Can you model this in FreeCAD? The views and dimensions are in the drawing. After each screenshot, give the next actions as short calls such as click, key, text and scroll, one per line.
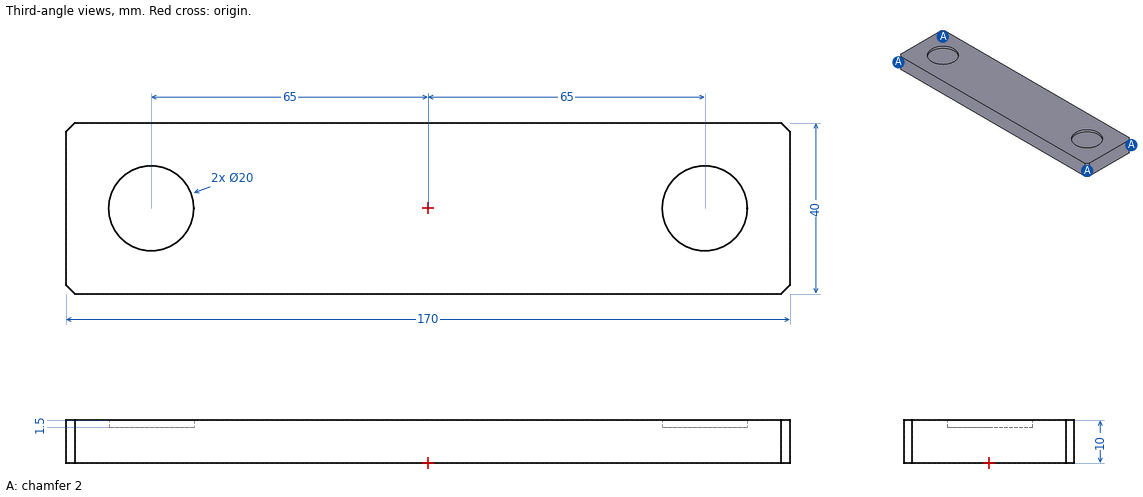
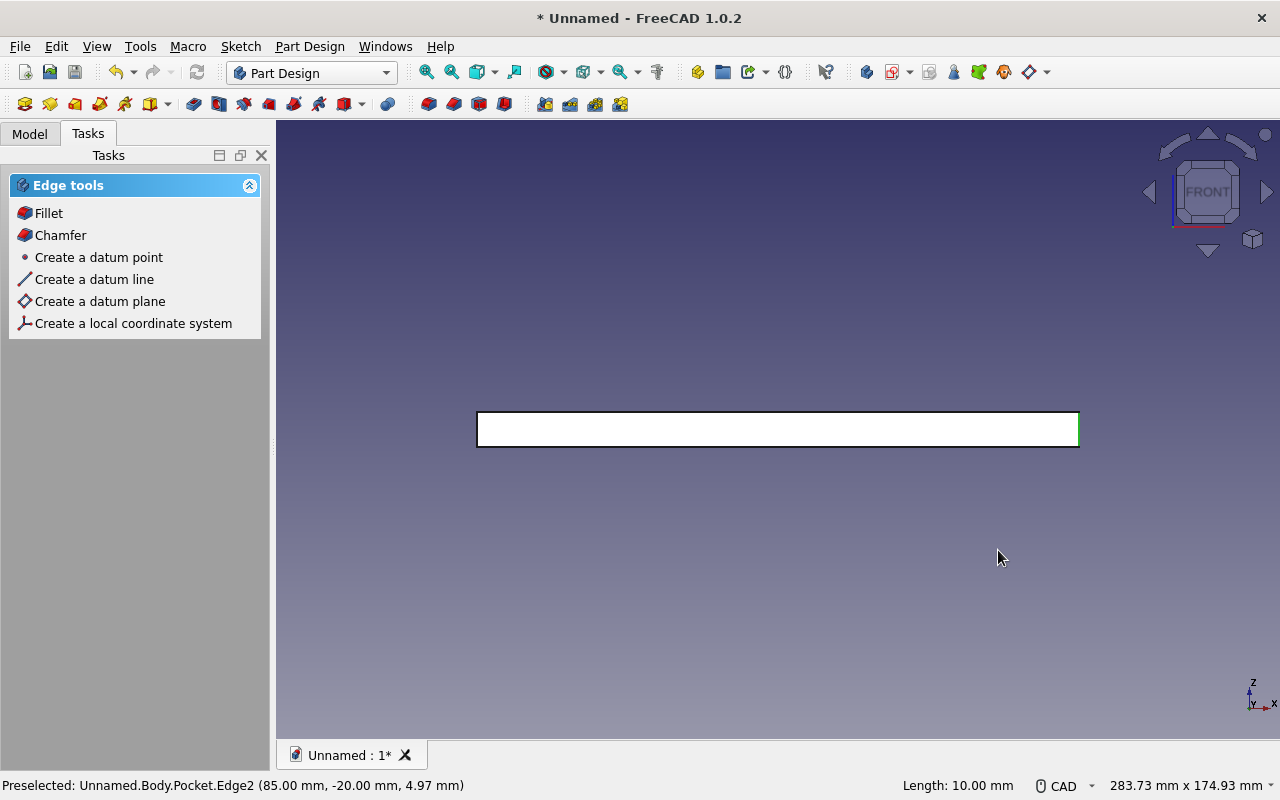
click(477, 428, ctrl)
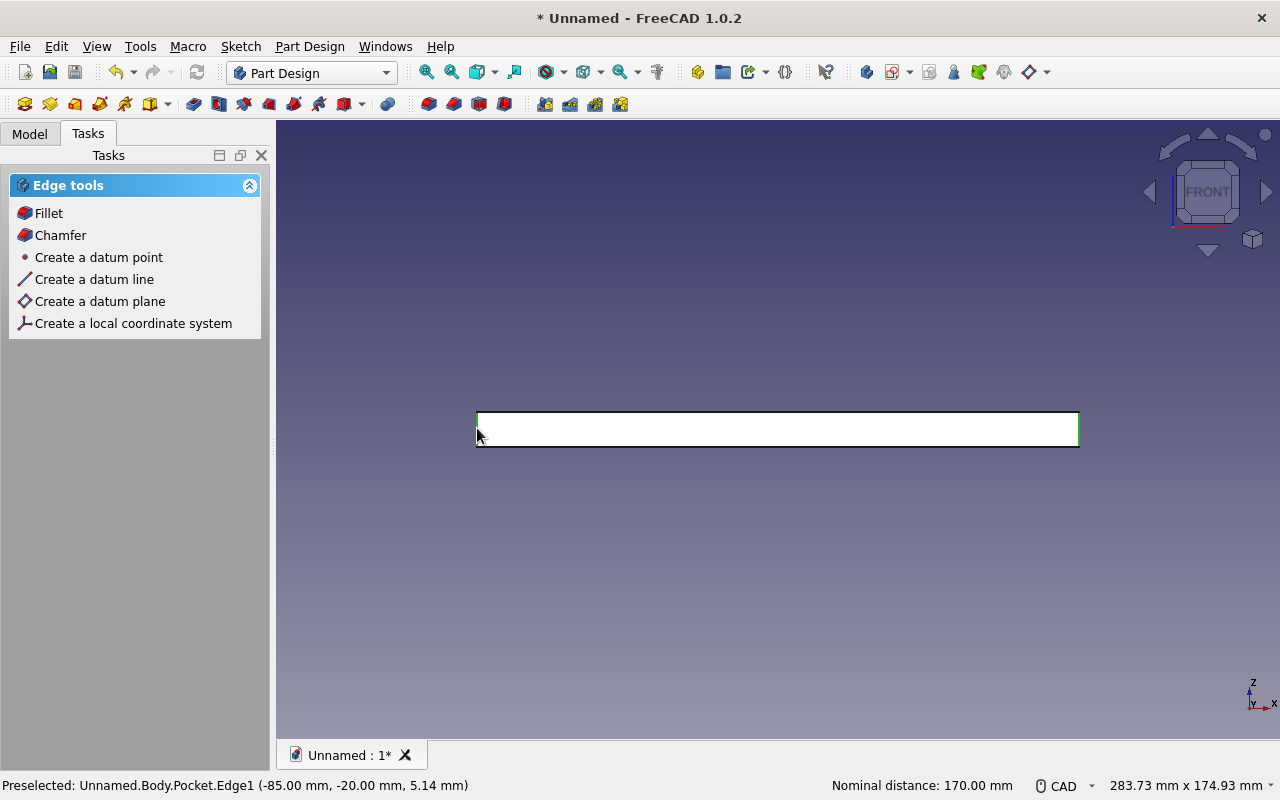
key(3)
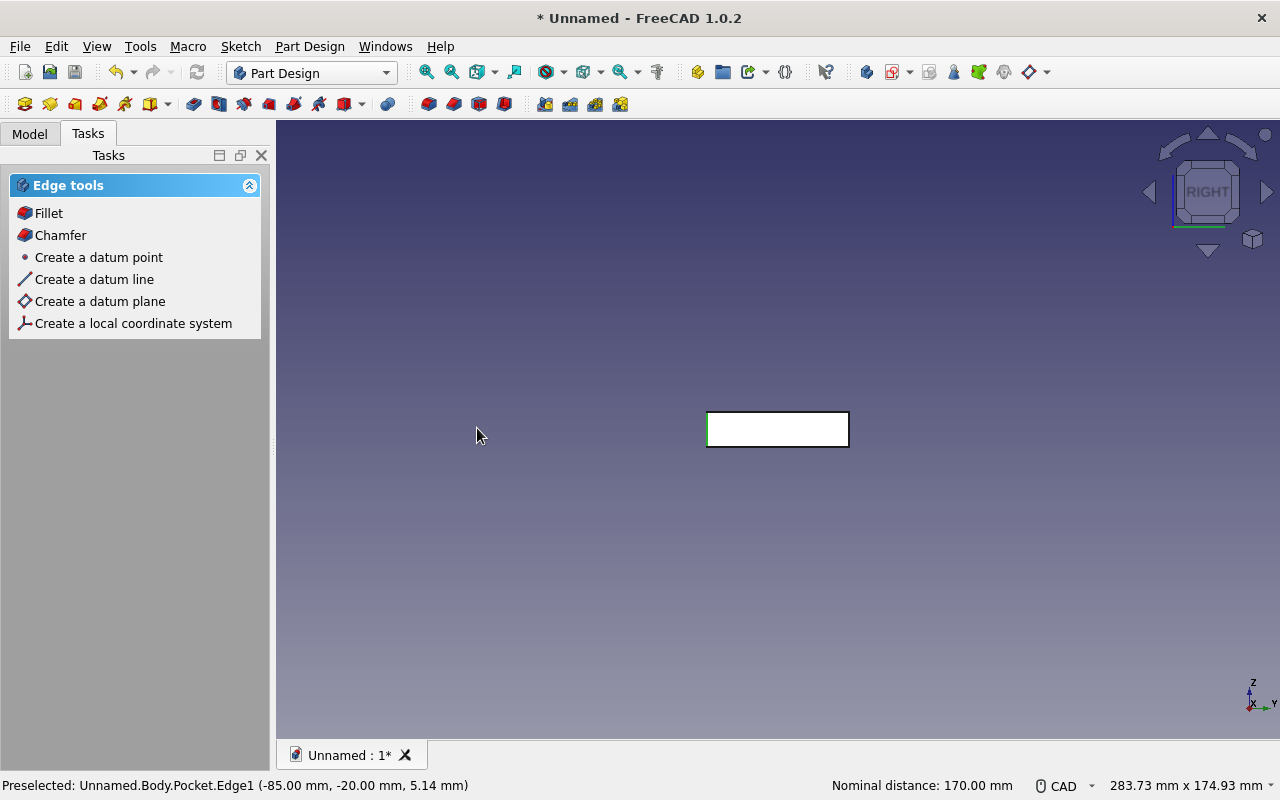
key(v)
key(f)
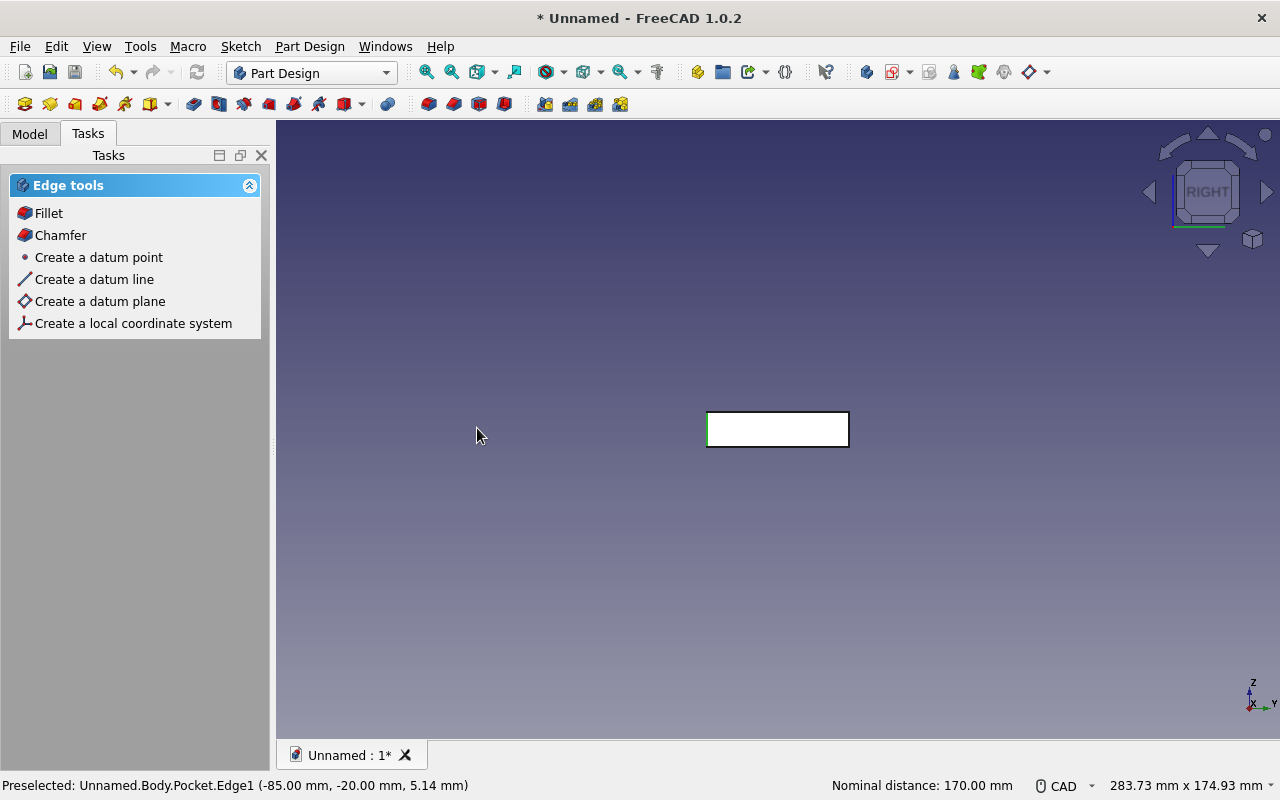
click(849, 428, ctrl)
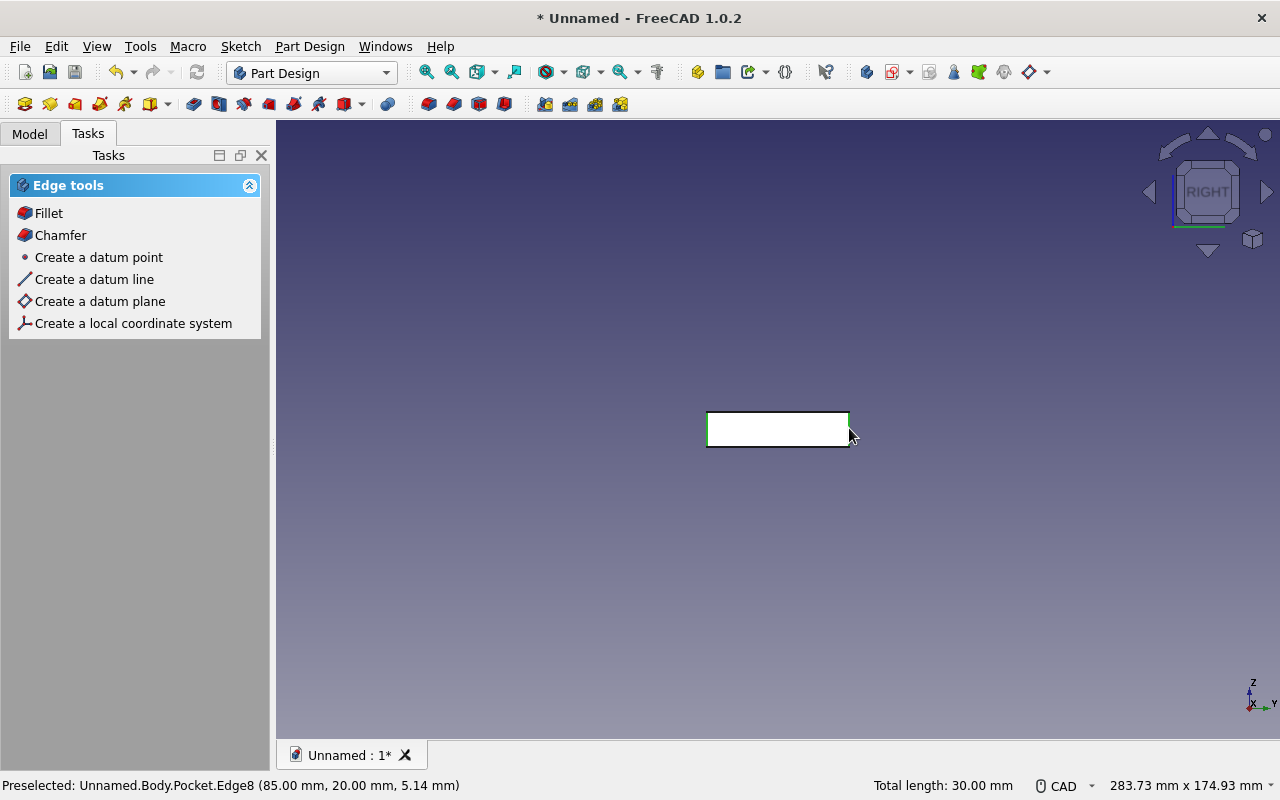
key(5)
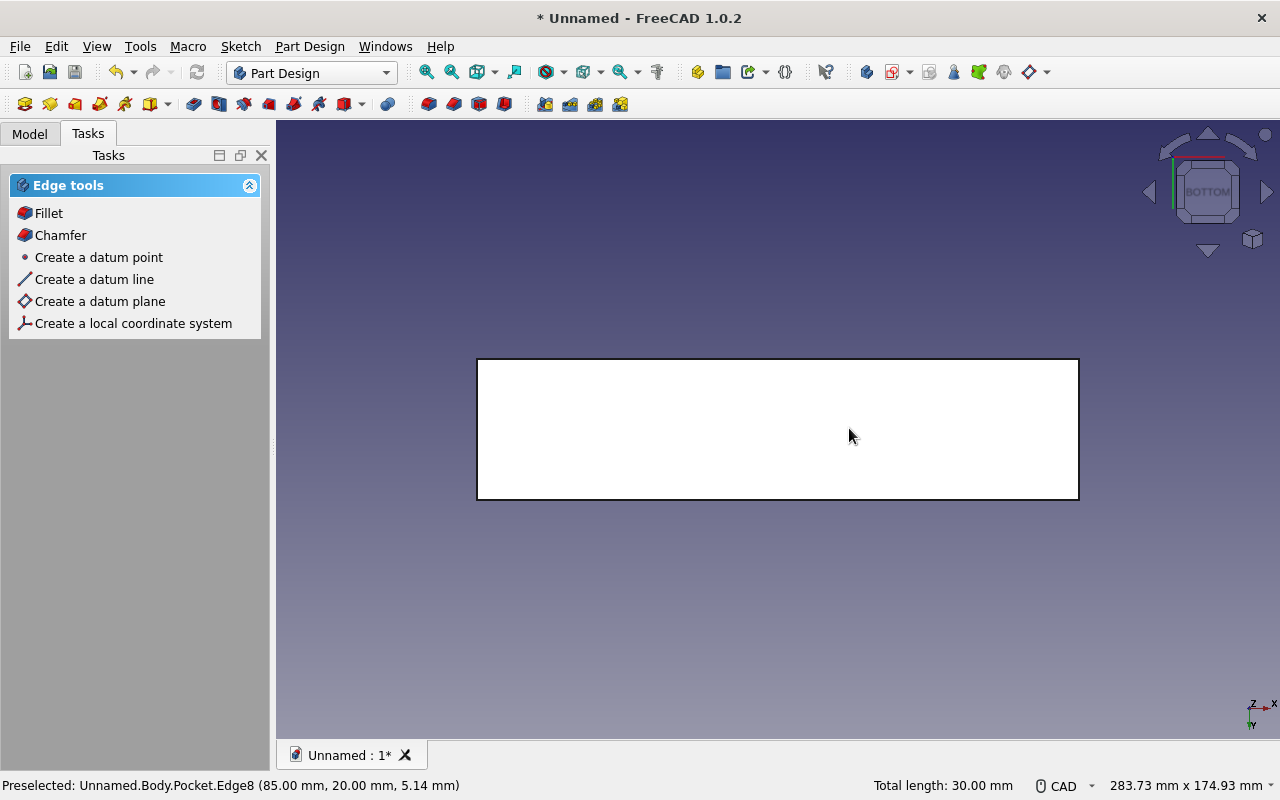
key(4)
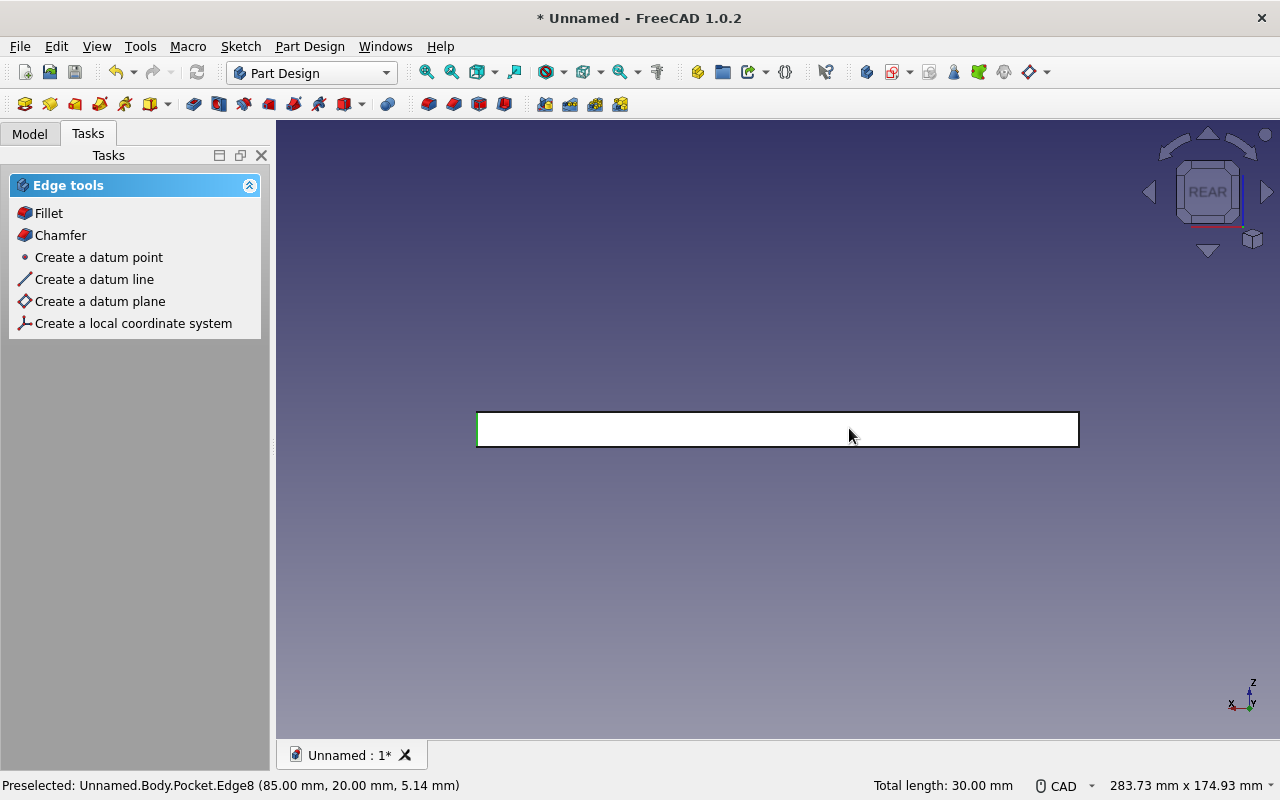
click(1079, 428, ctrl)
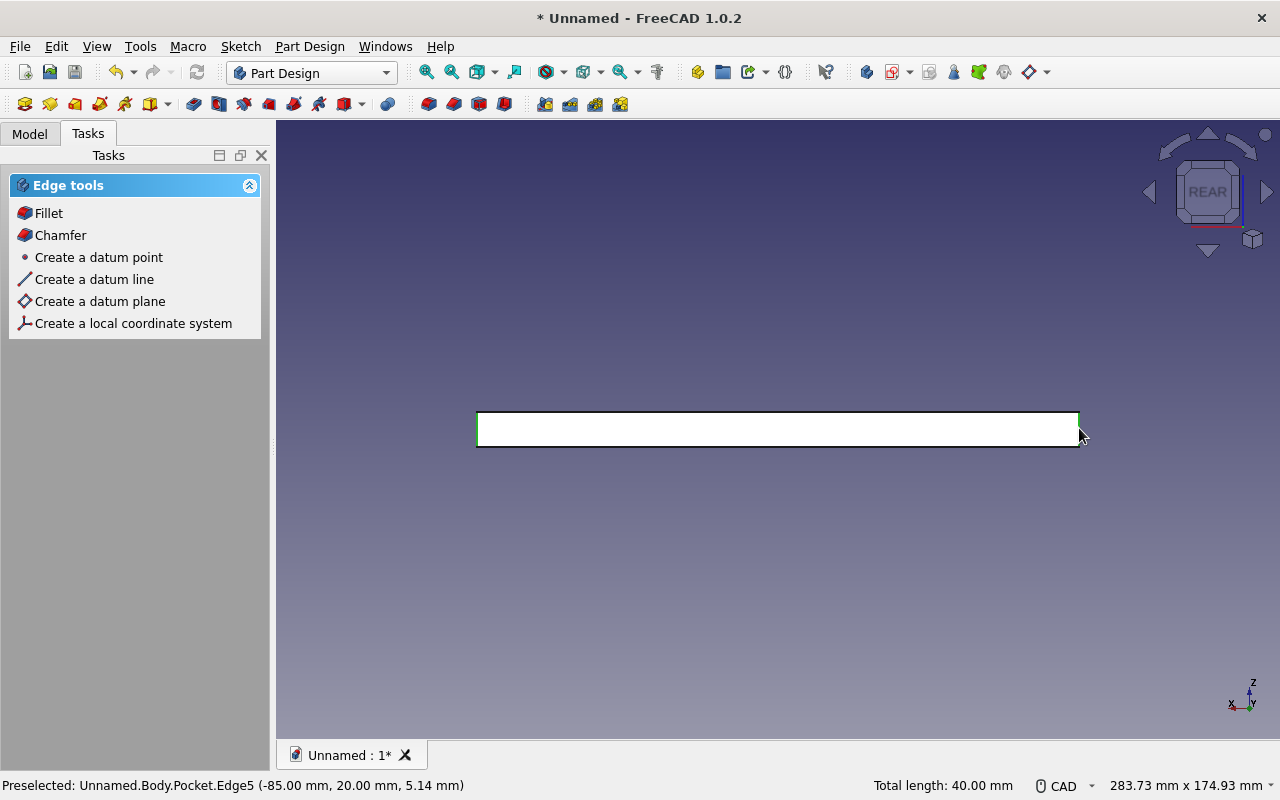
click(454, 104)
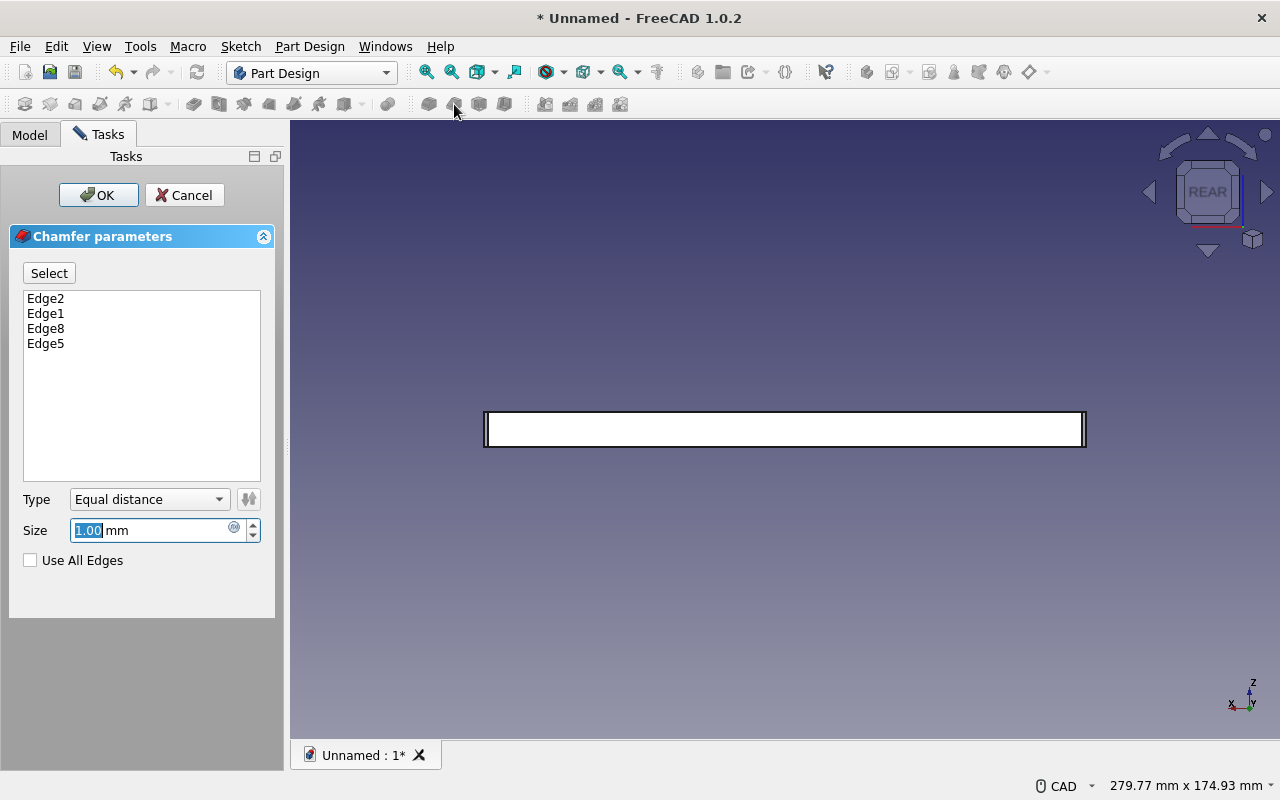
text(2)
key(Tab)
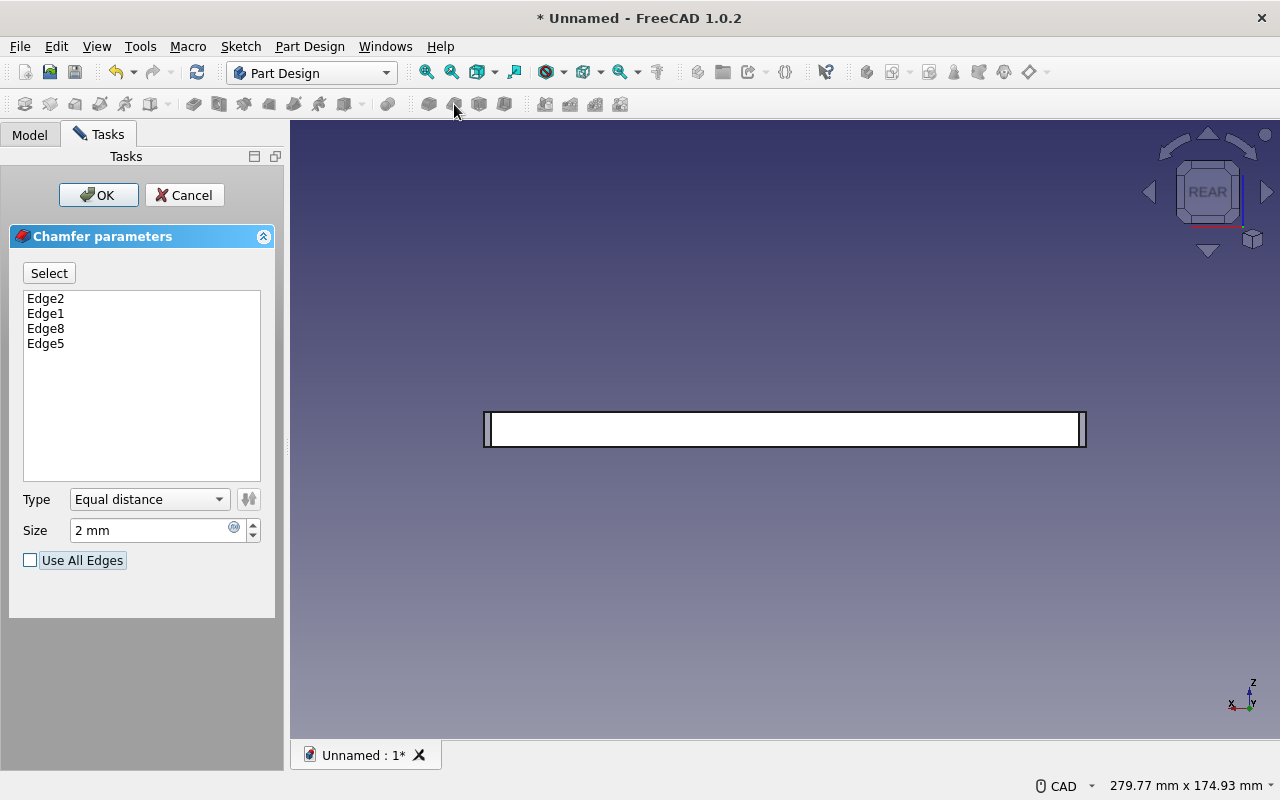
click(99, 195)